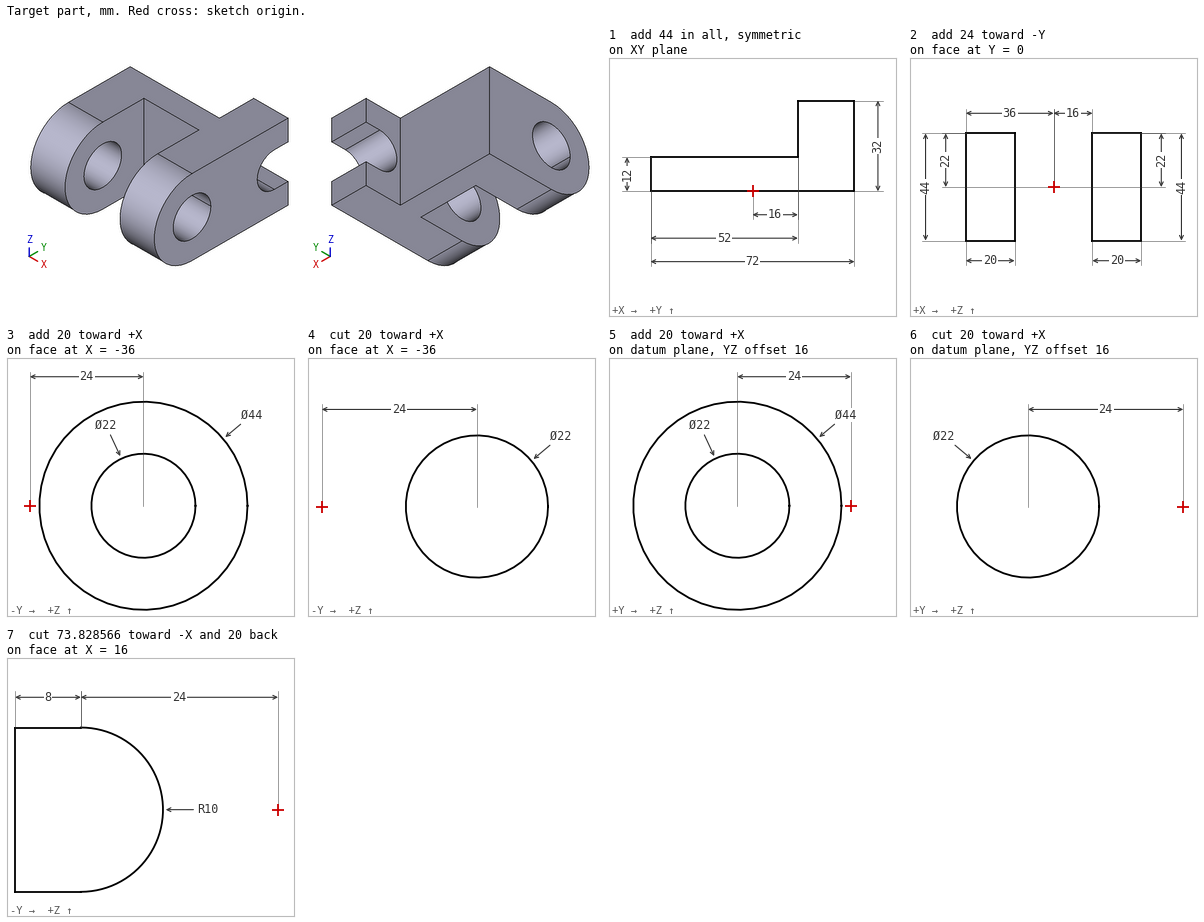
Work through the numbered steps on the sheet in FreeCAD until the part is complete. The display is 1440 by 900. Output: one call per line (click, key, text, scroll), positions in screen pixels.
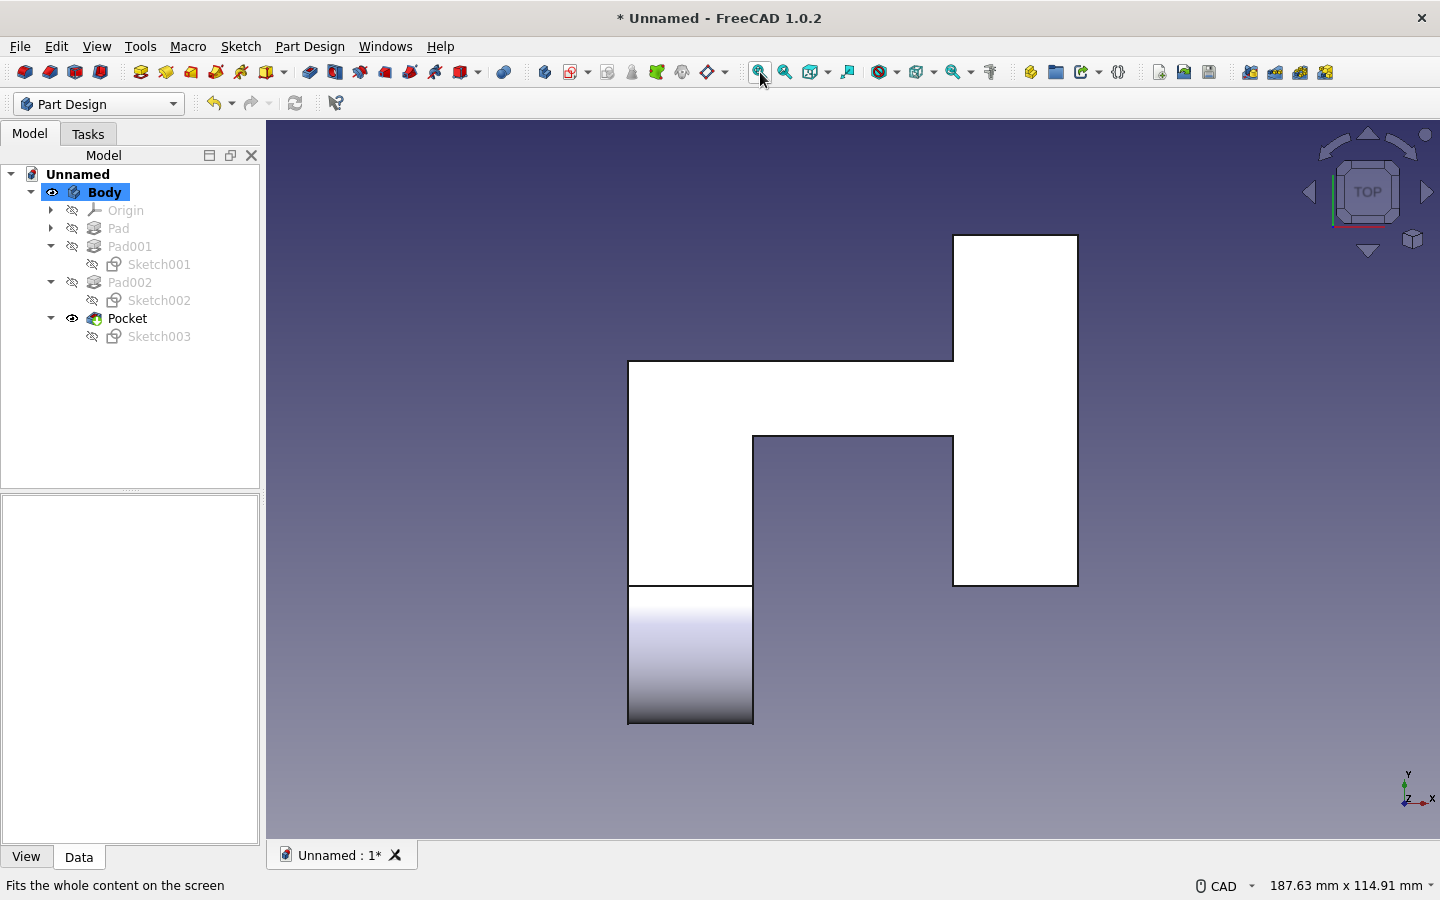
key(6)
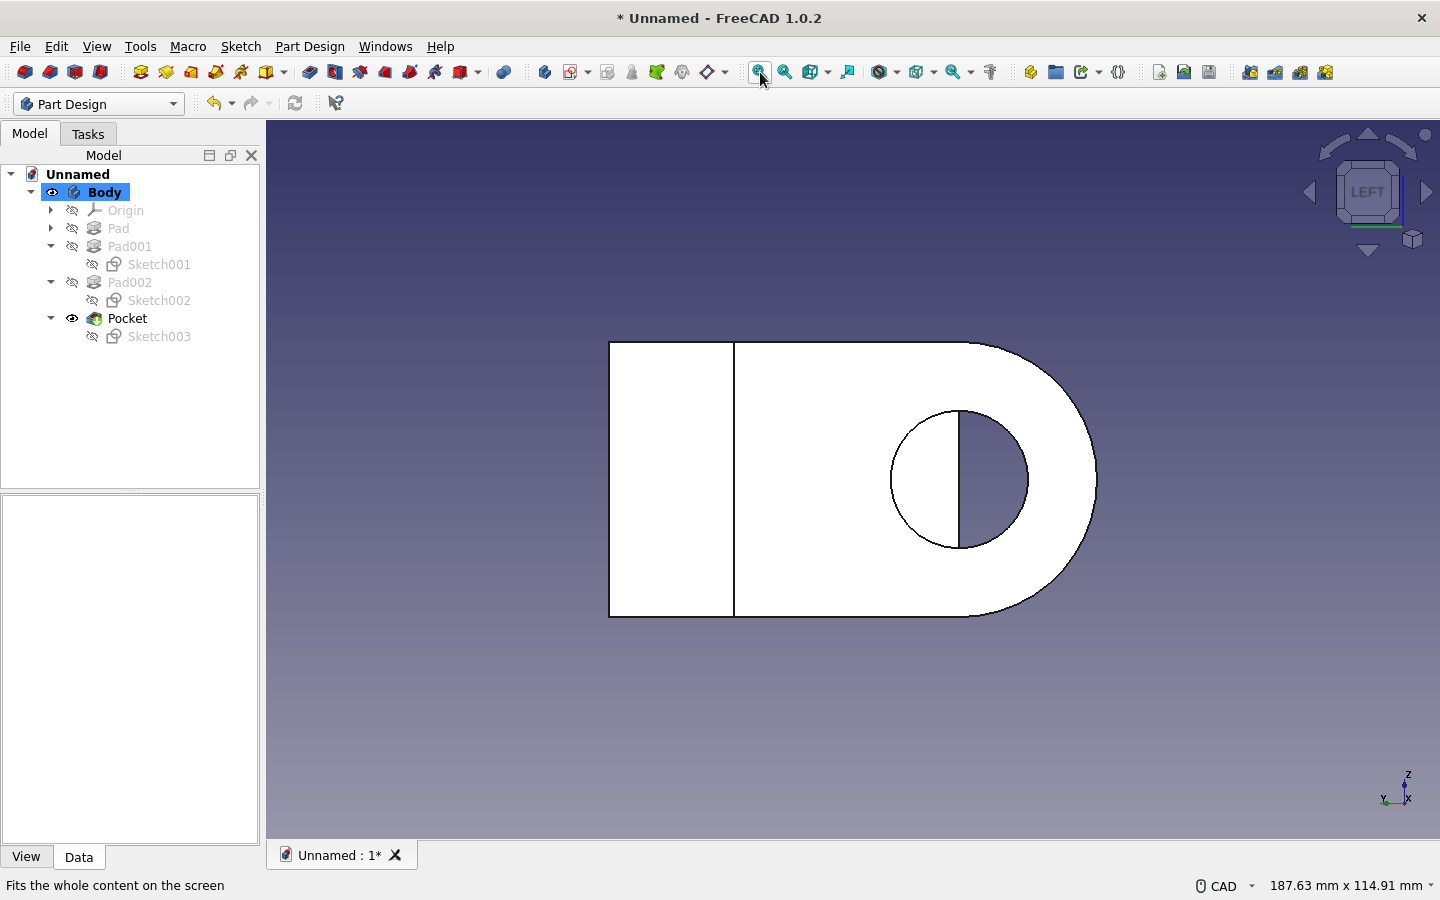
click(760, 72)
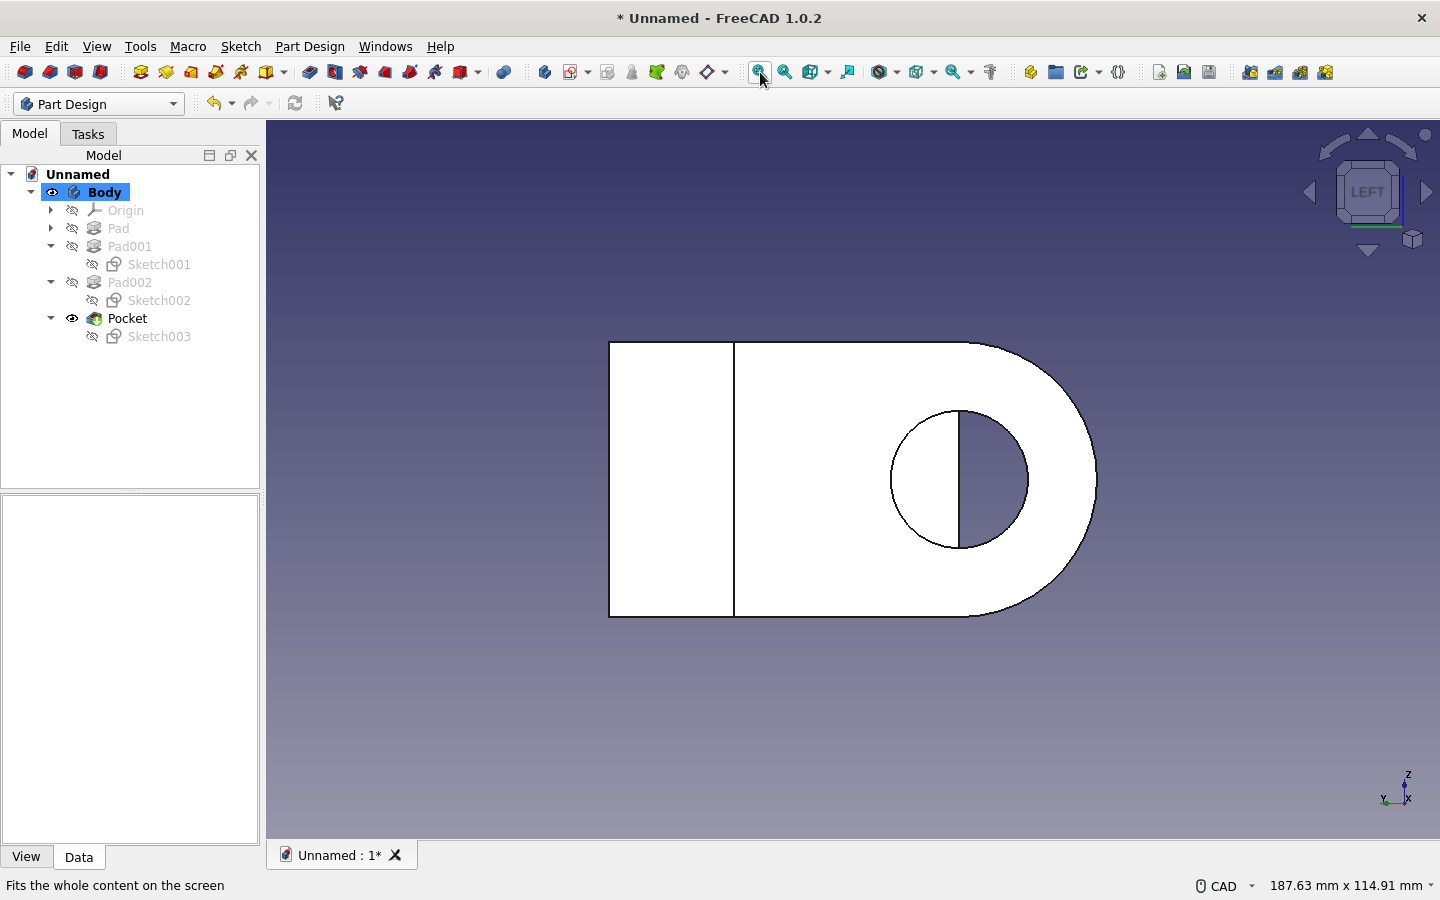
key(1)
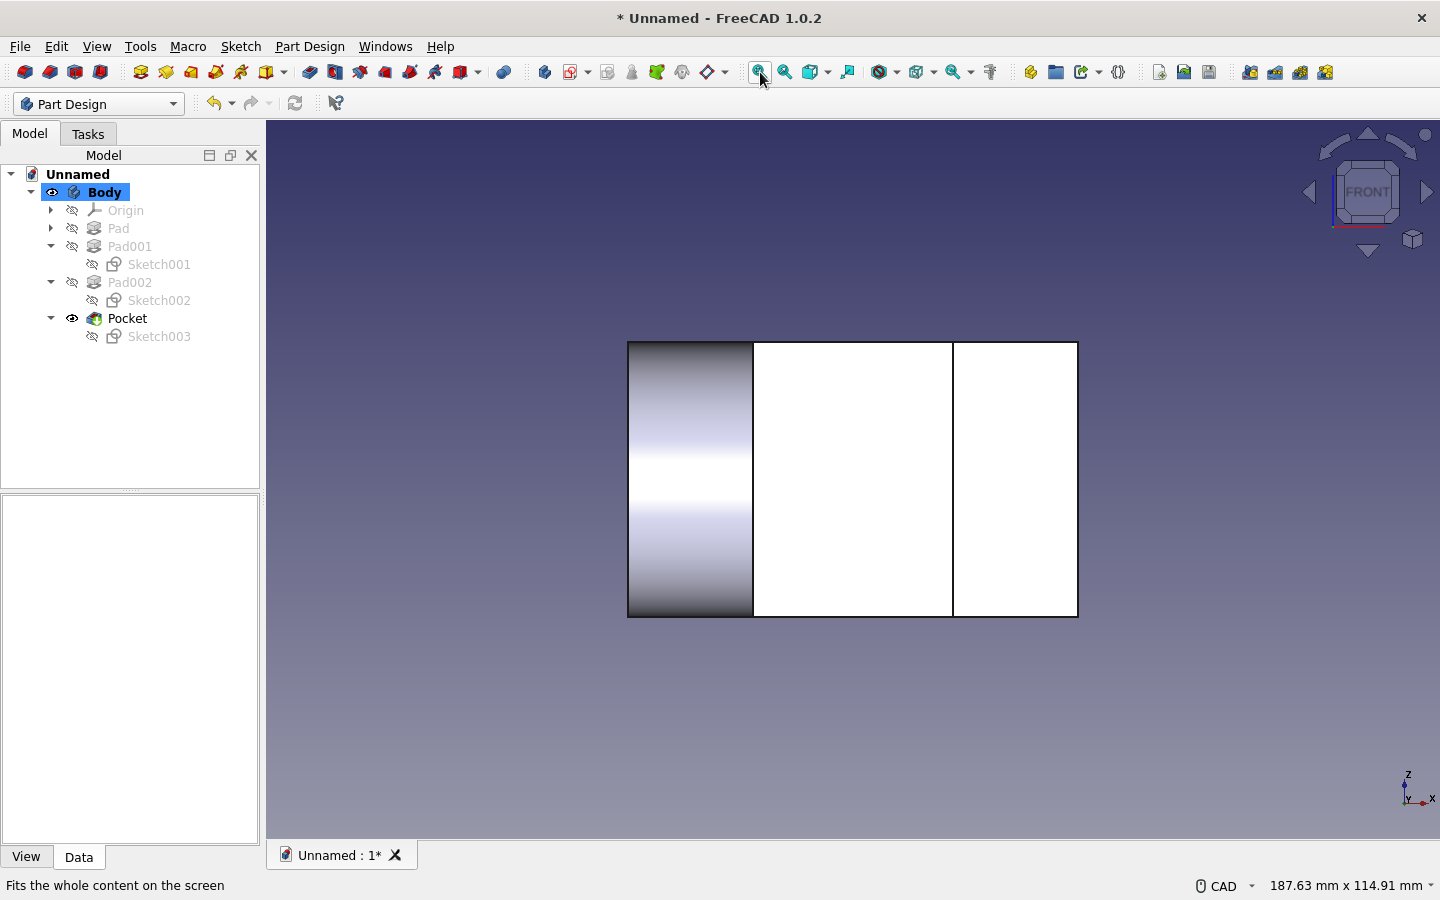
click(760, 72)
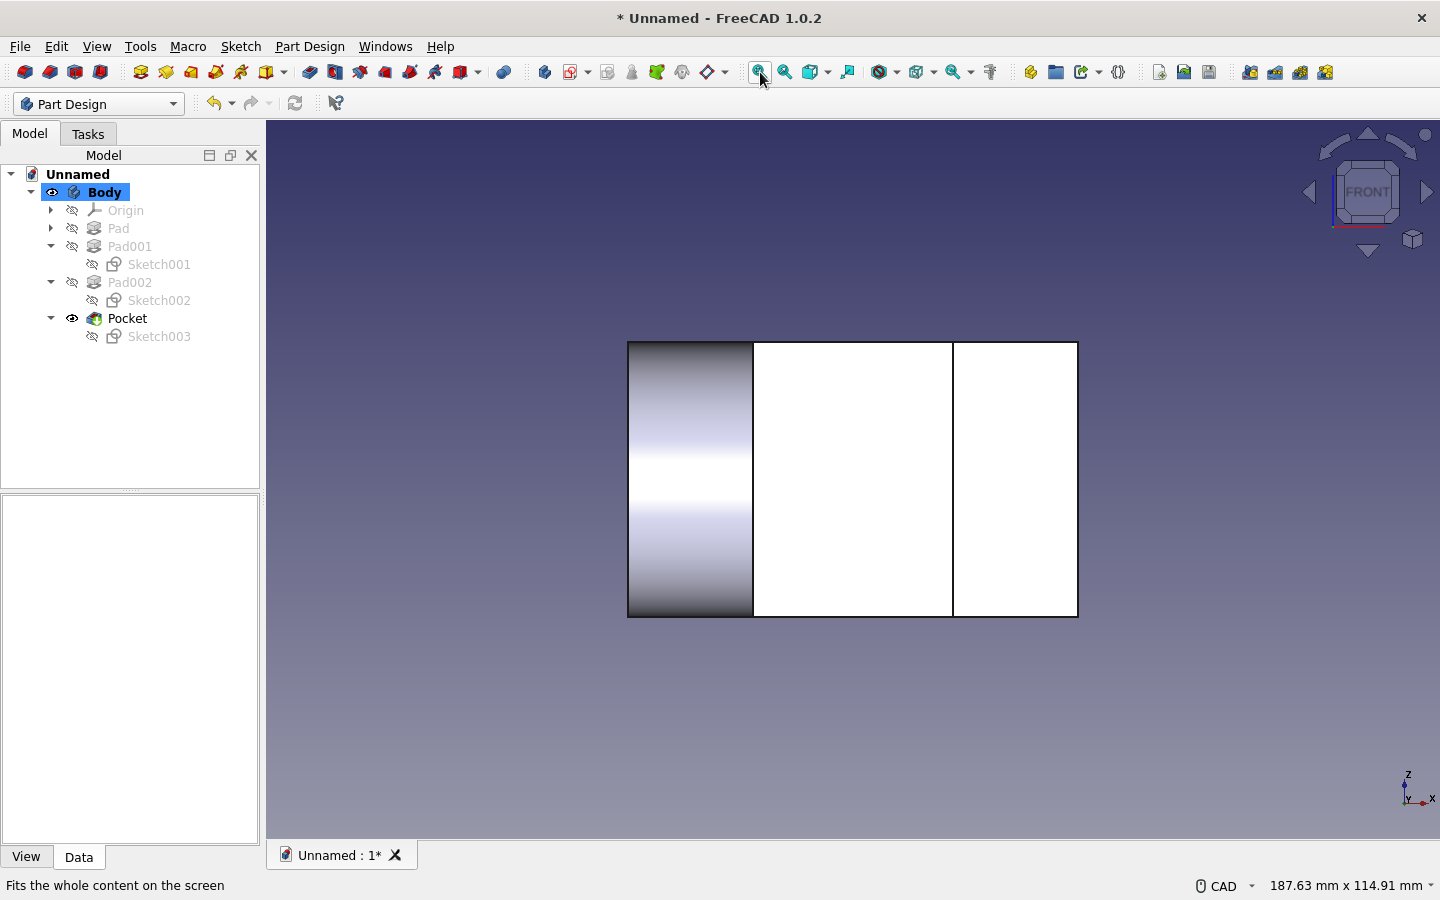
click(51, 210)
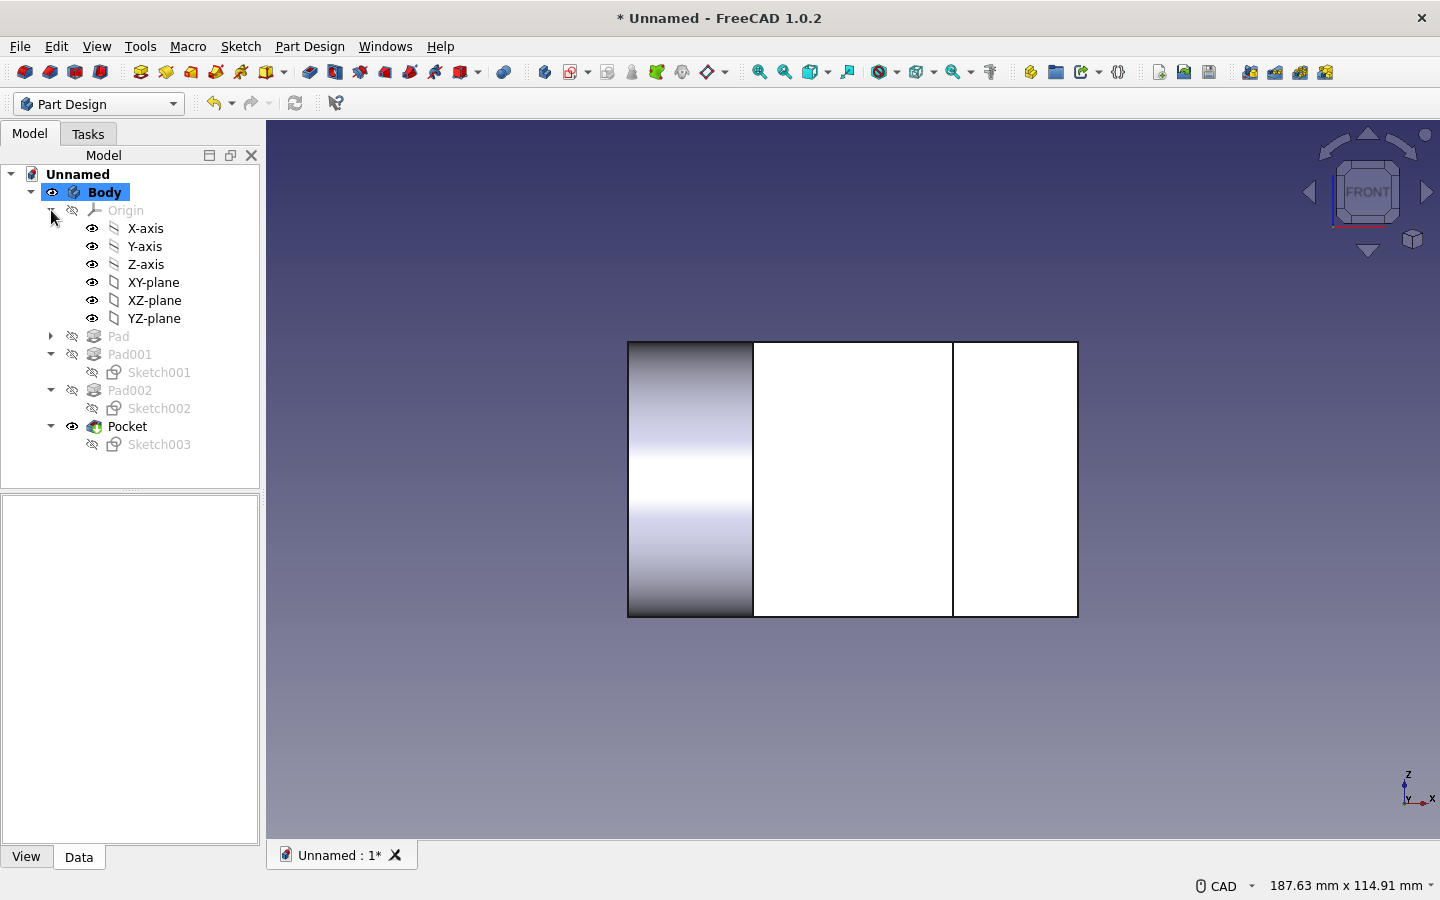
click(137, 318)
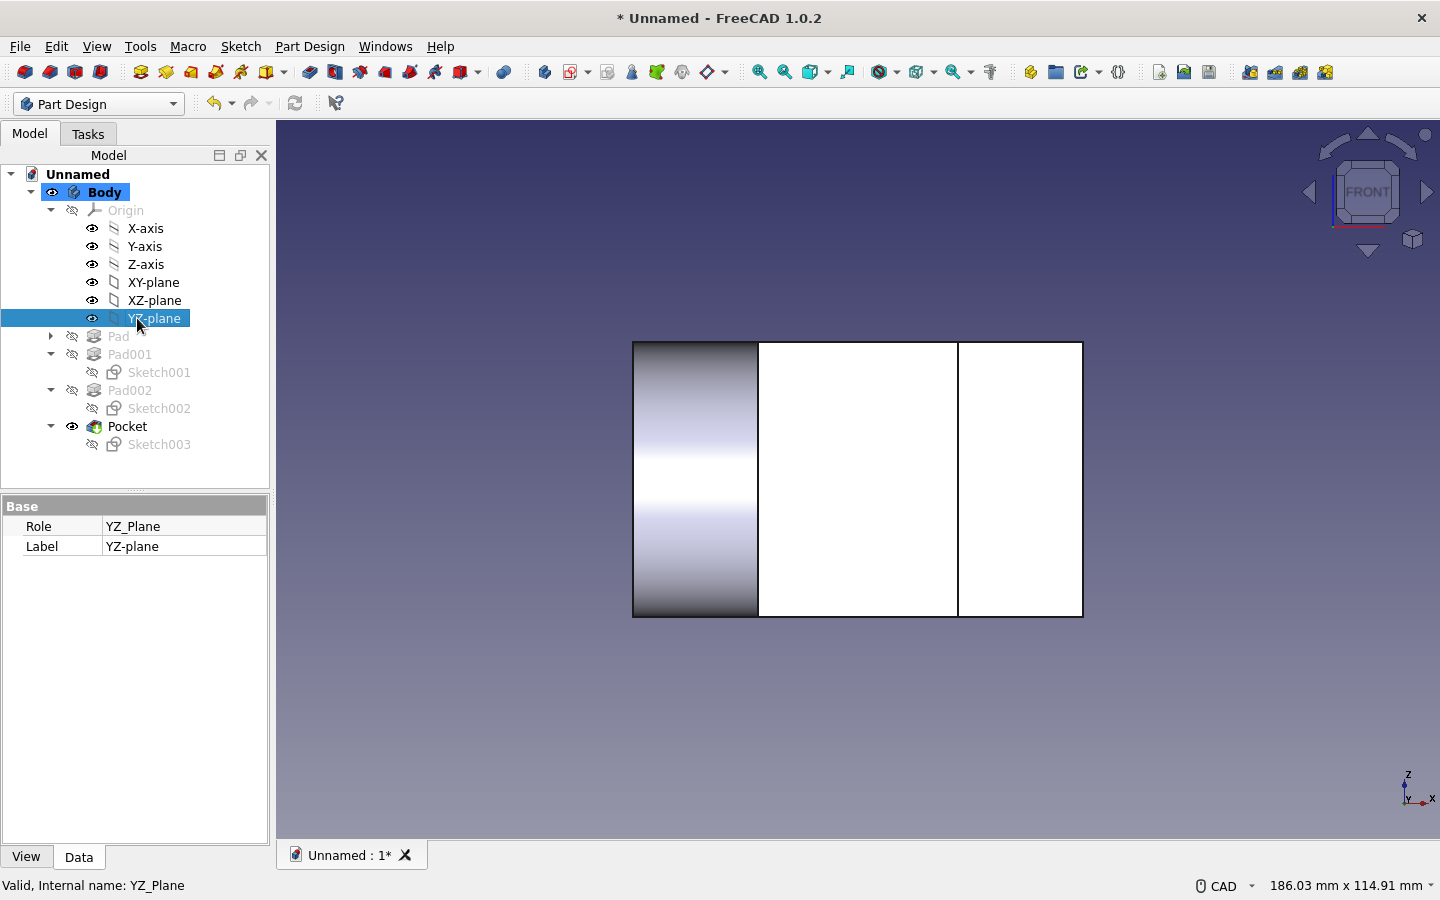
click(706, 72)